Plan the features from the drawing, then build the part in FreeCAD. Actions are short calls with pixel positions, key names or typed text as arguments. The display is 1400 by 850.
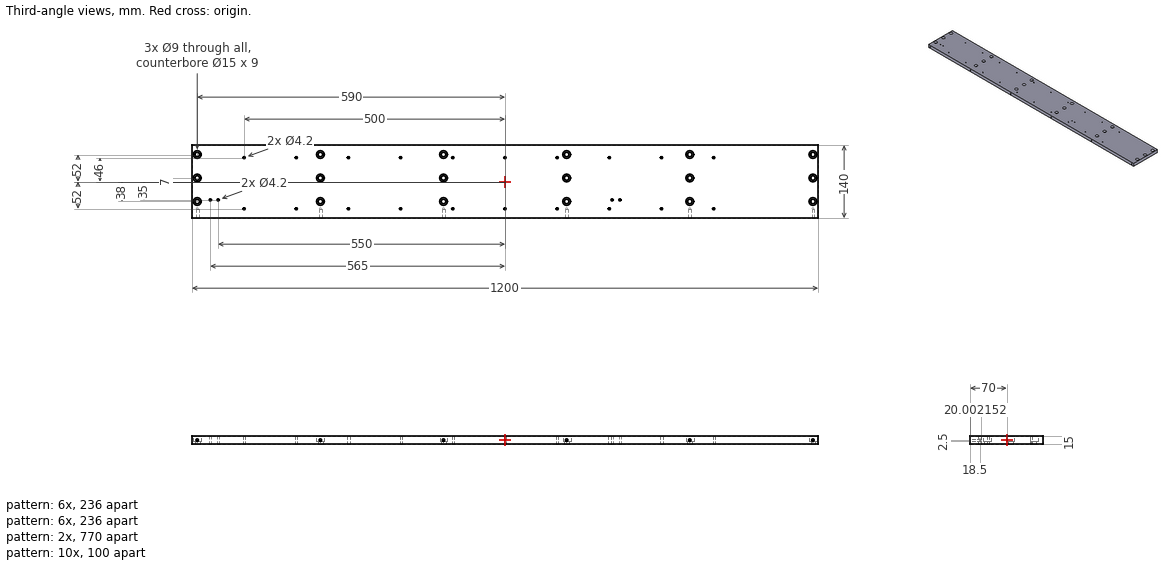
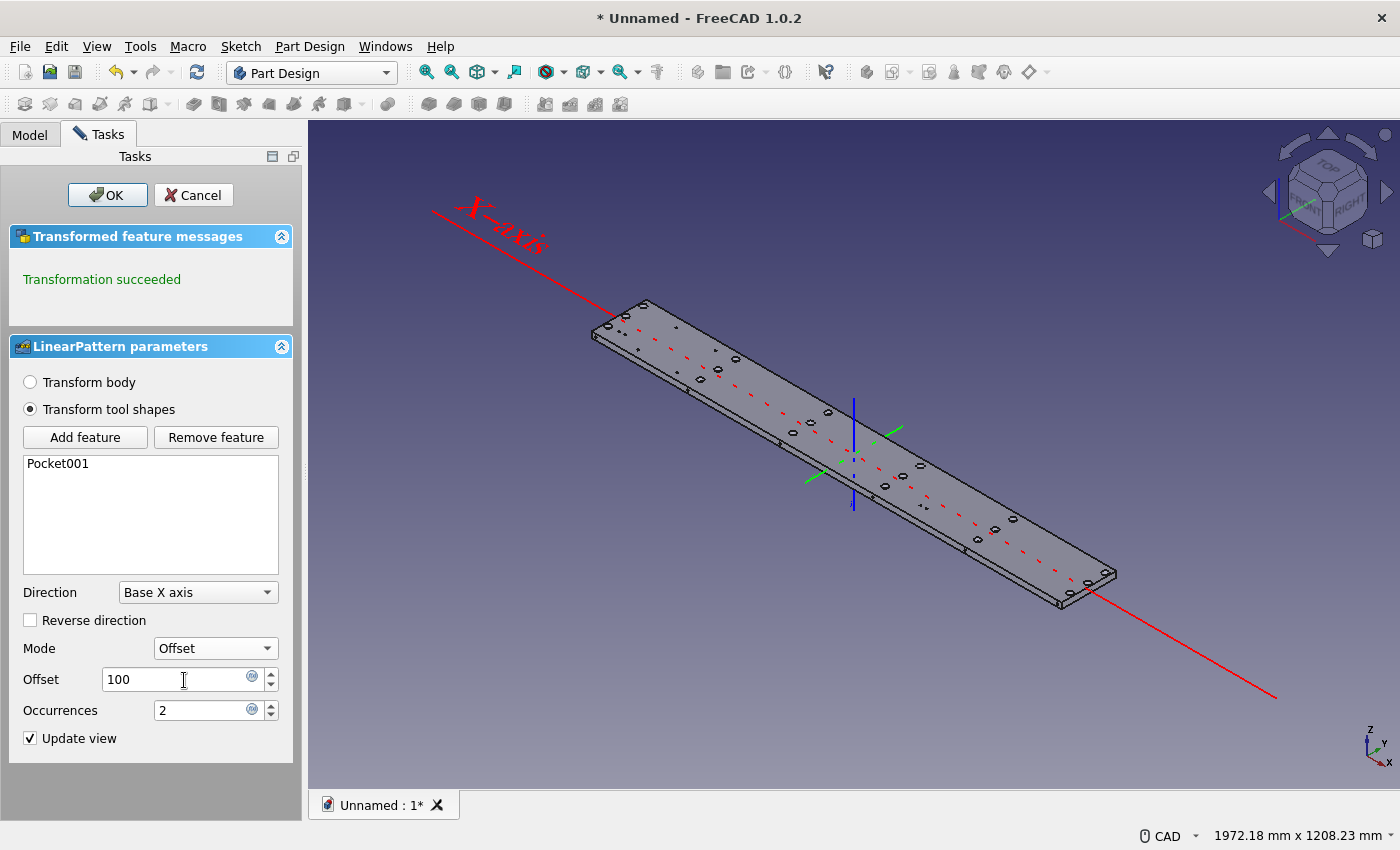
triple_click(210, 710)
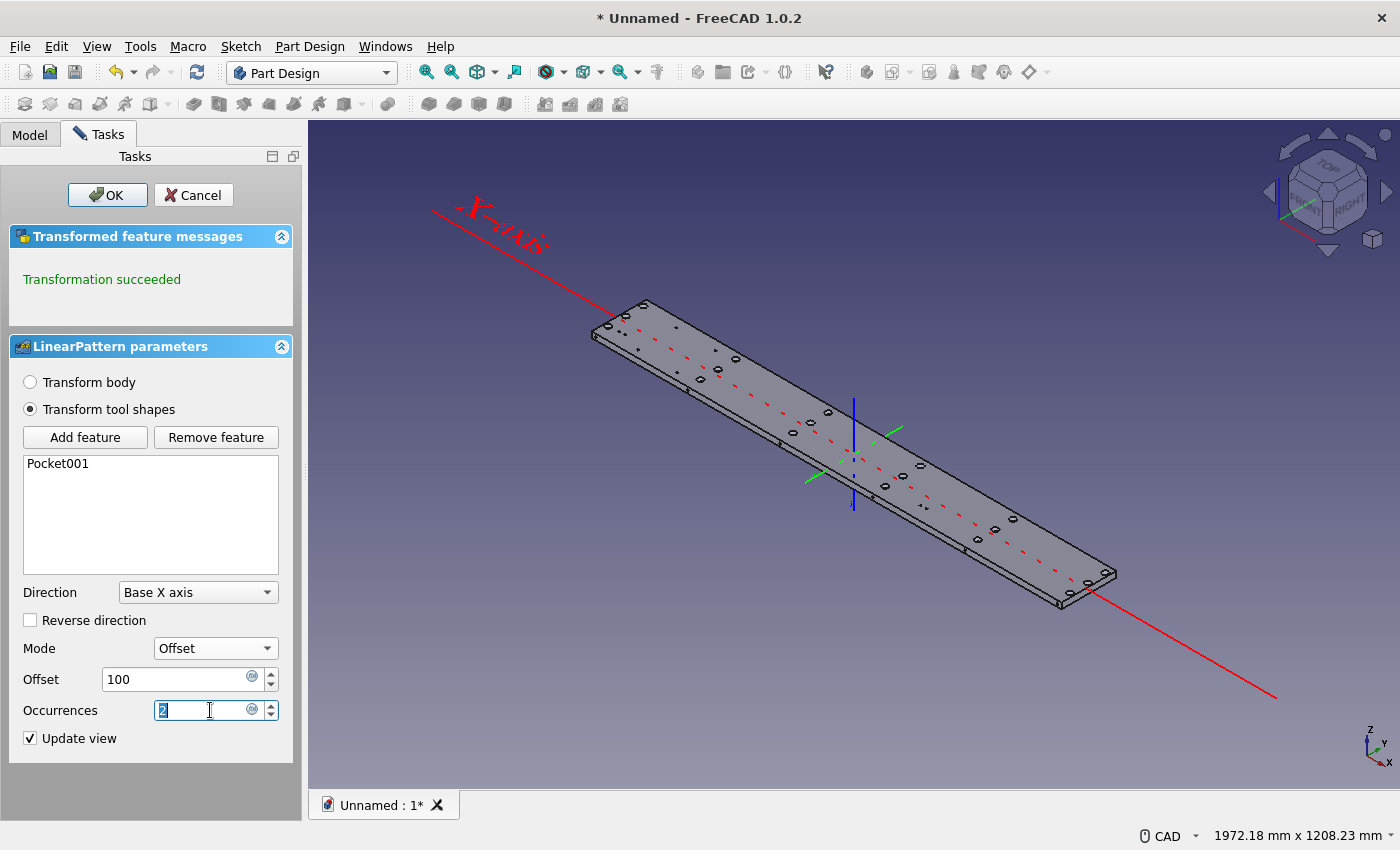
text(10)
key(Tab)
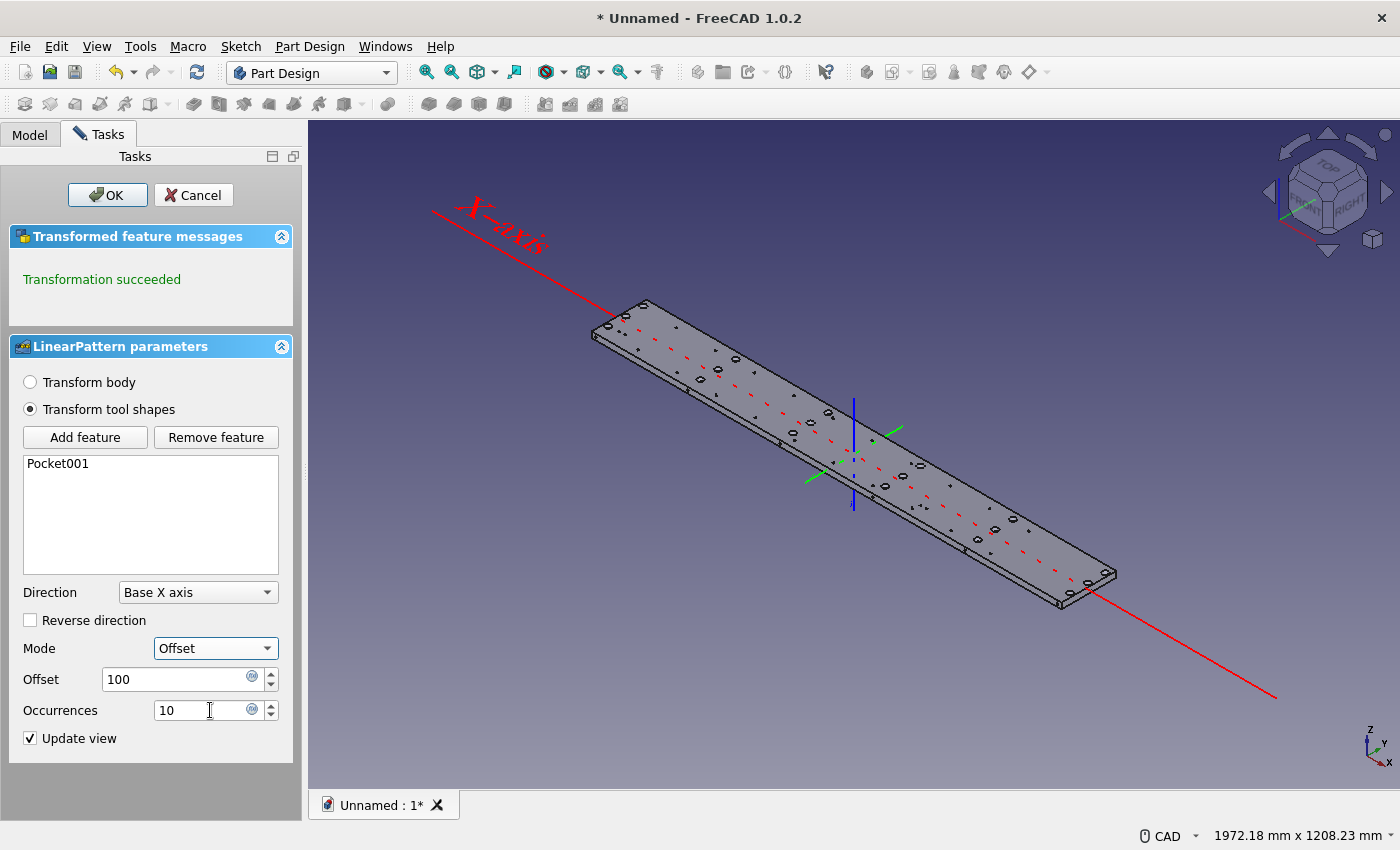
click(108, 195)